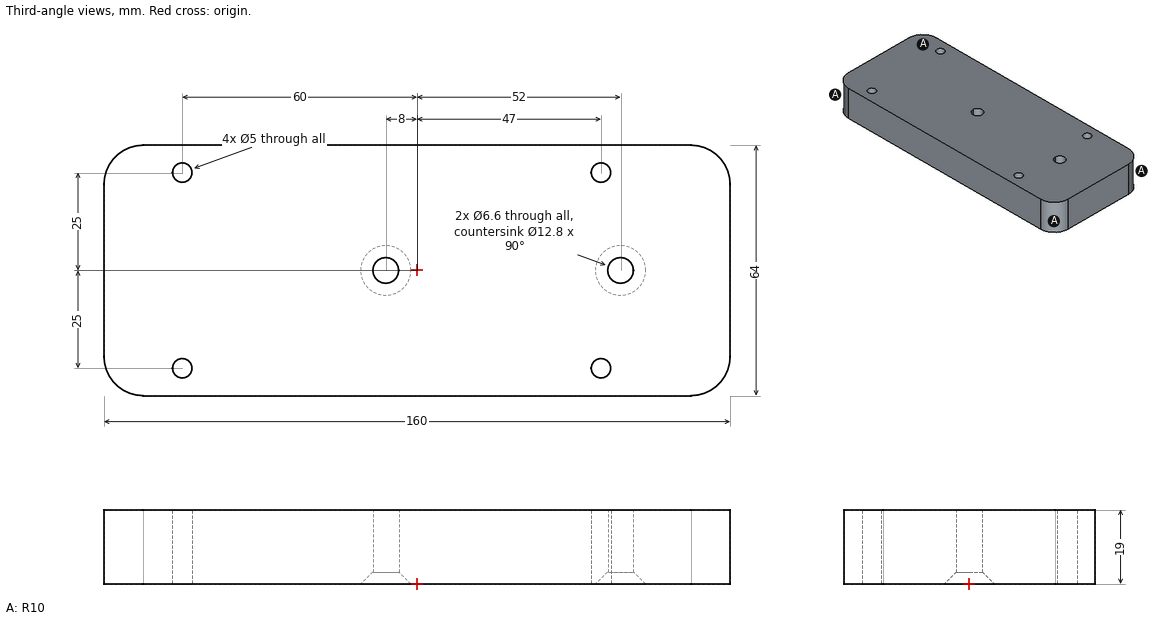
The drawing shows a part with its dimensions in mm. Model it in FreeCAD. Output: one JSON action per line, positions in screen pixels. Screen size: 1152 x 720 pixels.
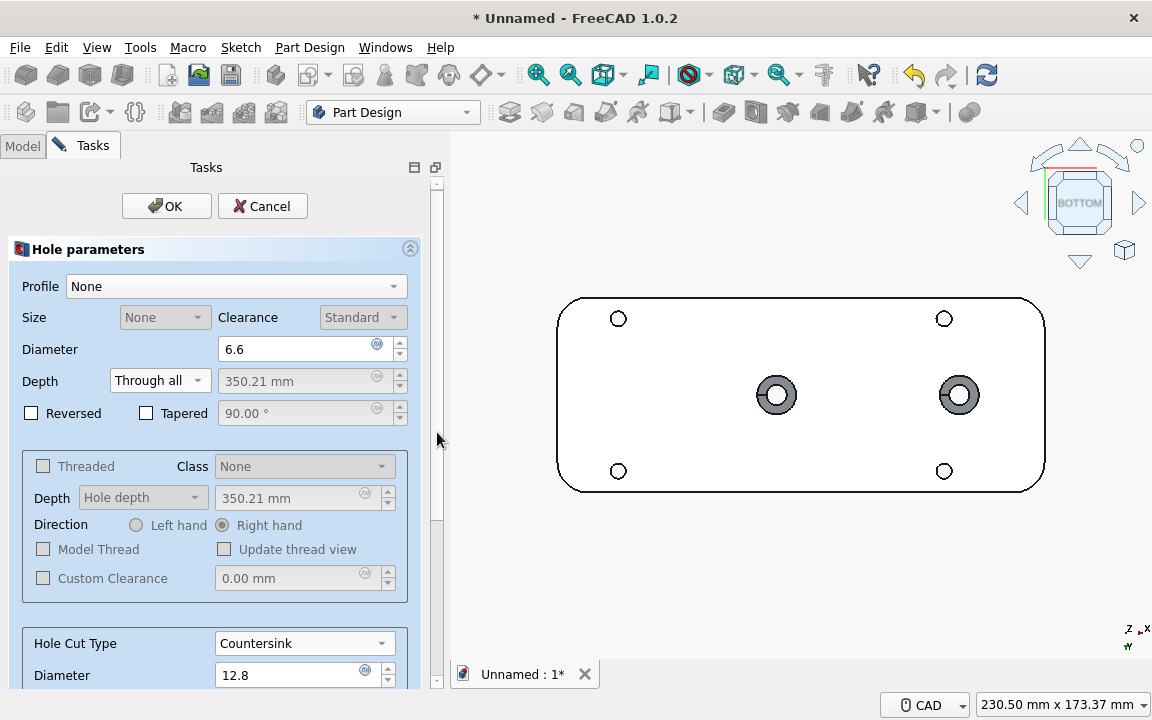
{"action": "left_click", "coordinate": [167, 206]}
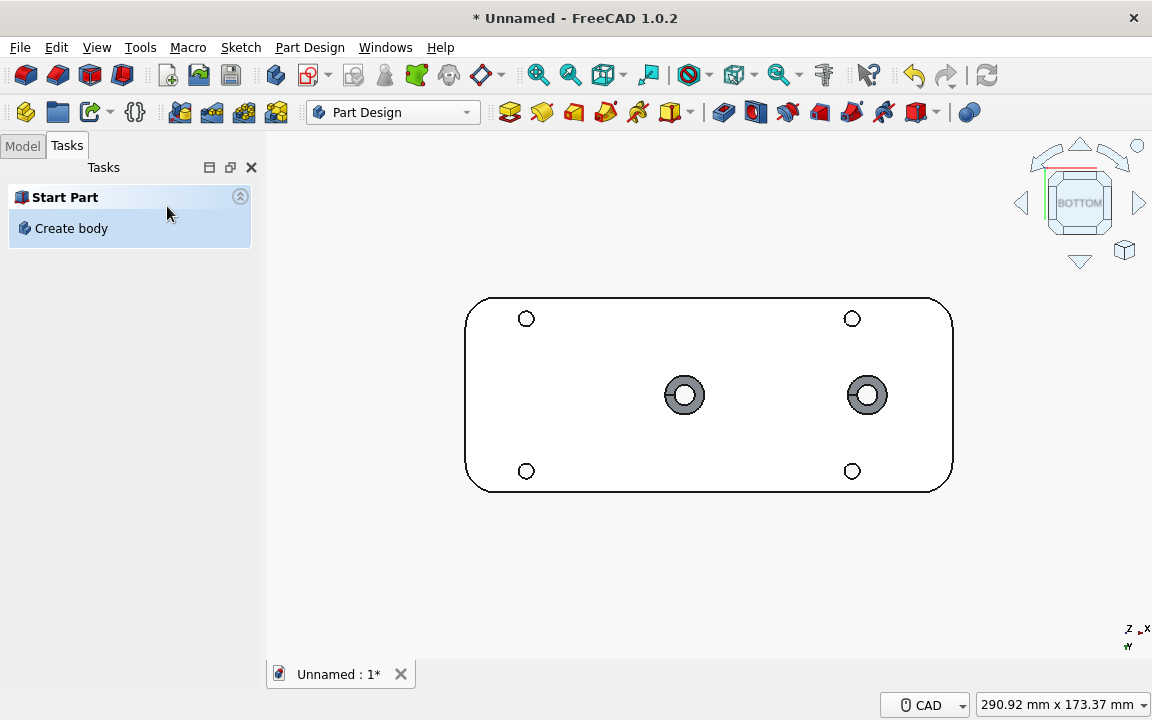
{"action": "key", "text": "0"}